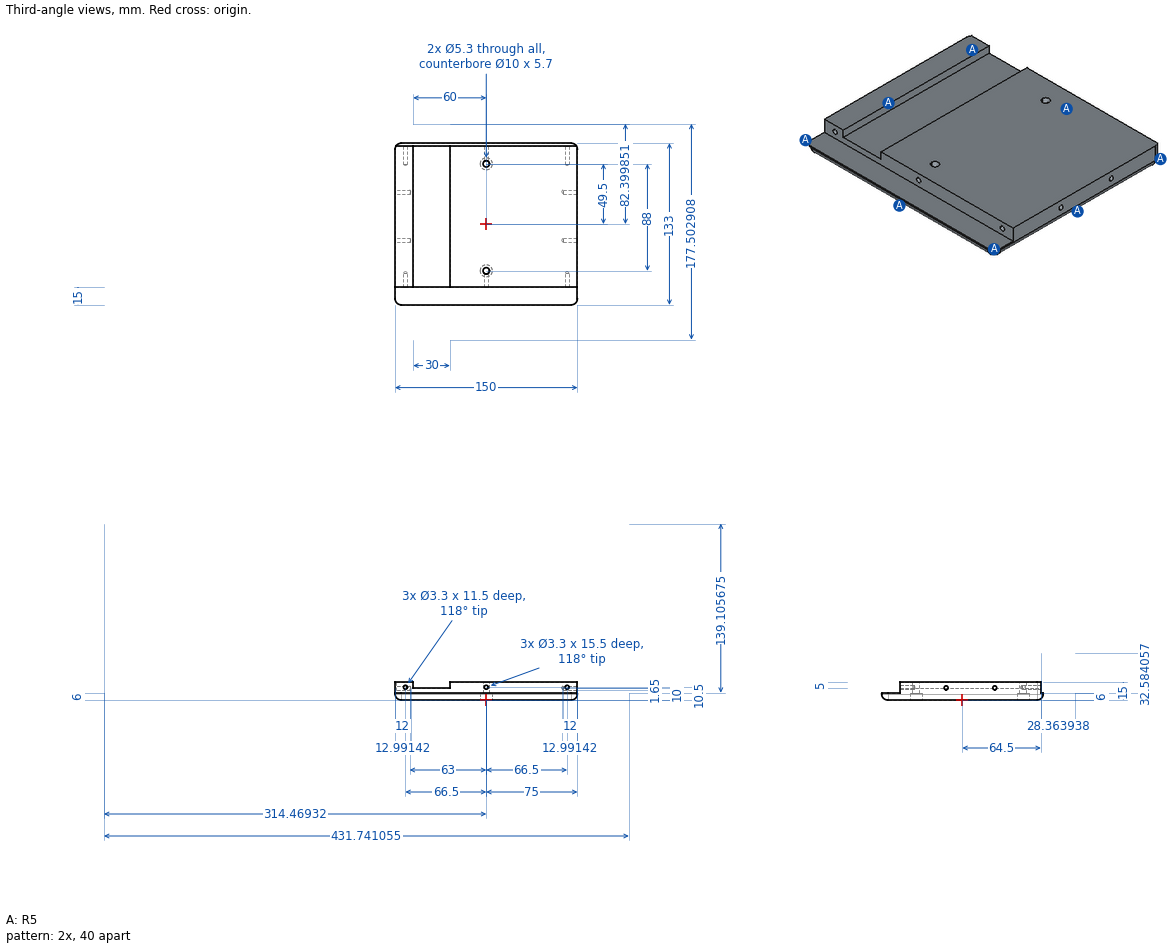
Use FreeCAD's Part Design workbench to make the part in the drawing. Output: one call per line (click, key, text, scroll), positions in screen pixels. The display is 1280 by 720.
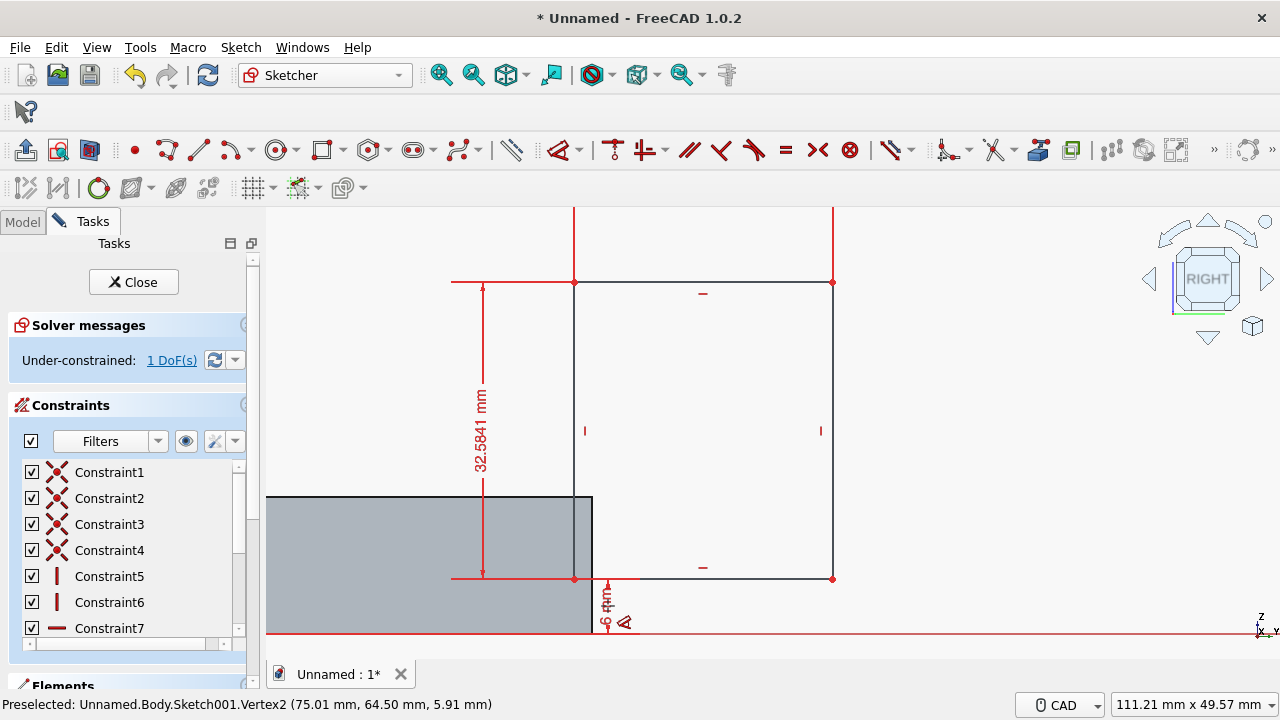
click(574, 282)
click(434, 248)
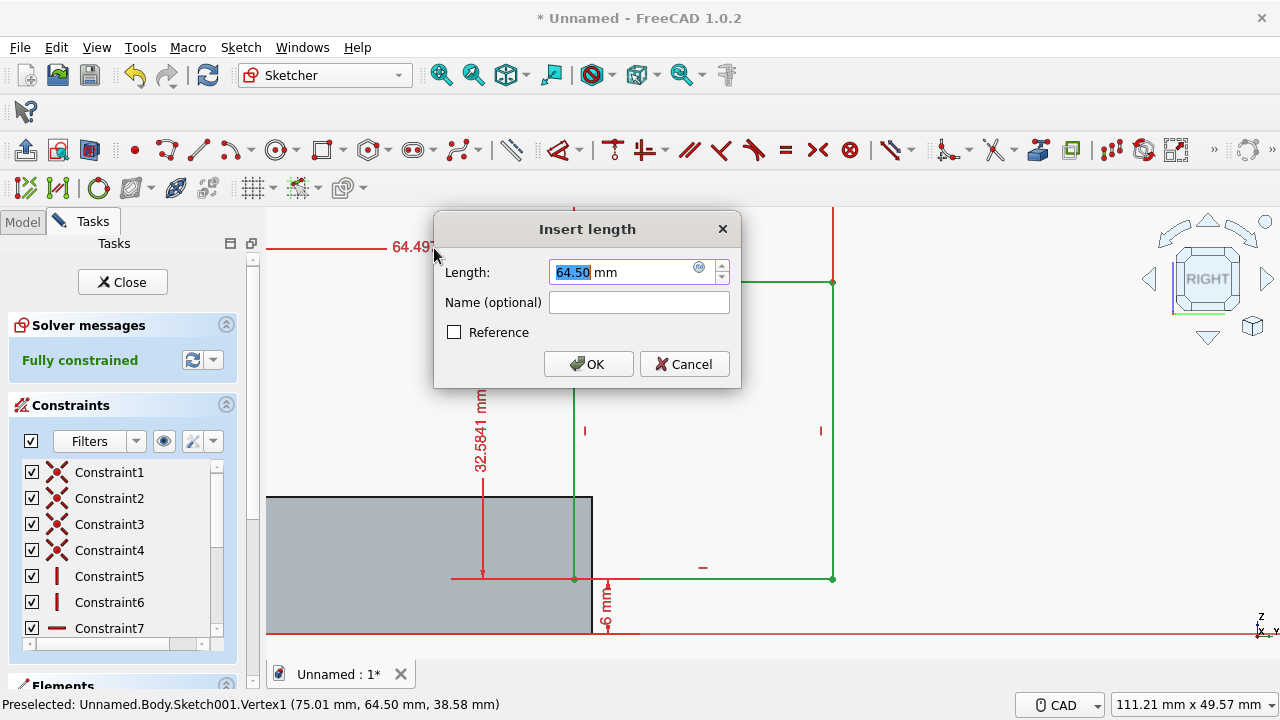
text(64.5)
key(Return)
key(Escape)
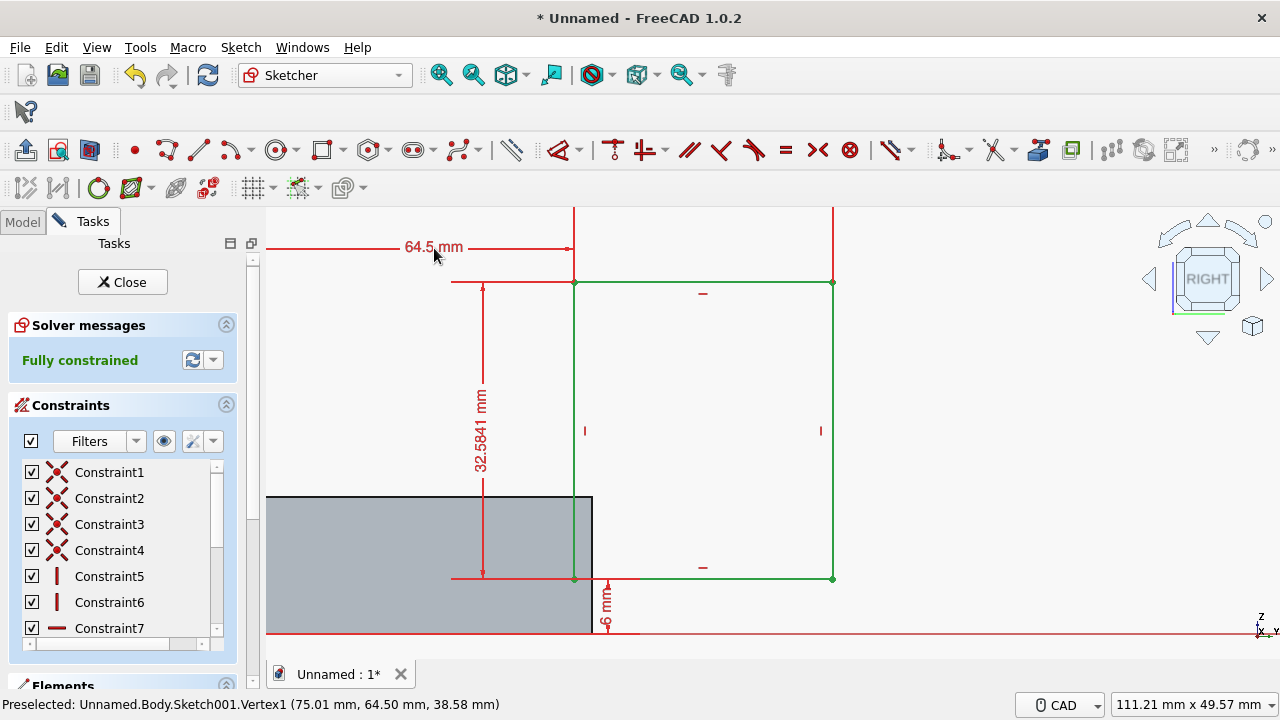
click(123, 282)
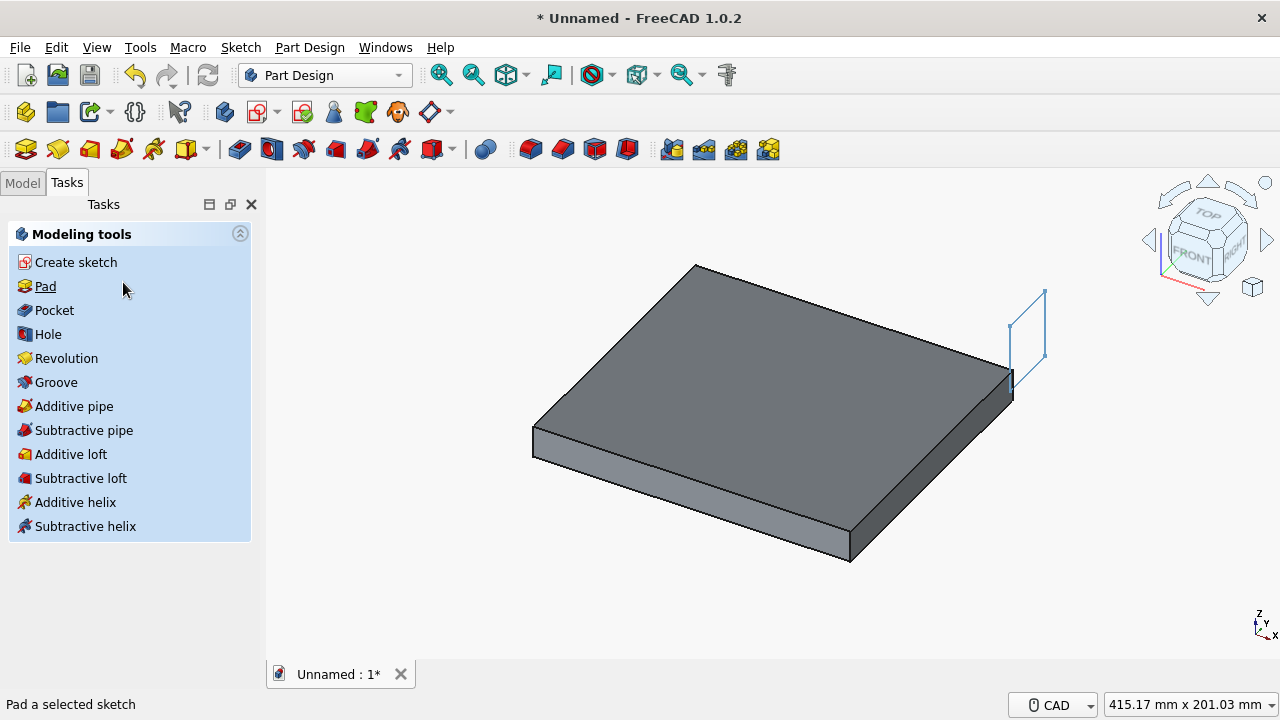
click(240, 150)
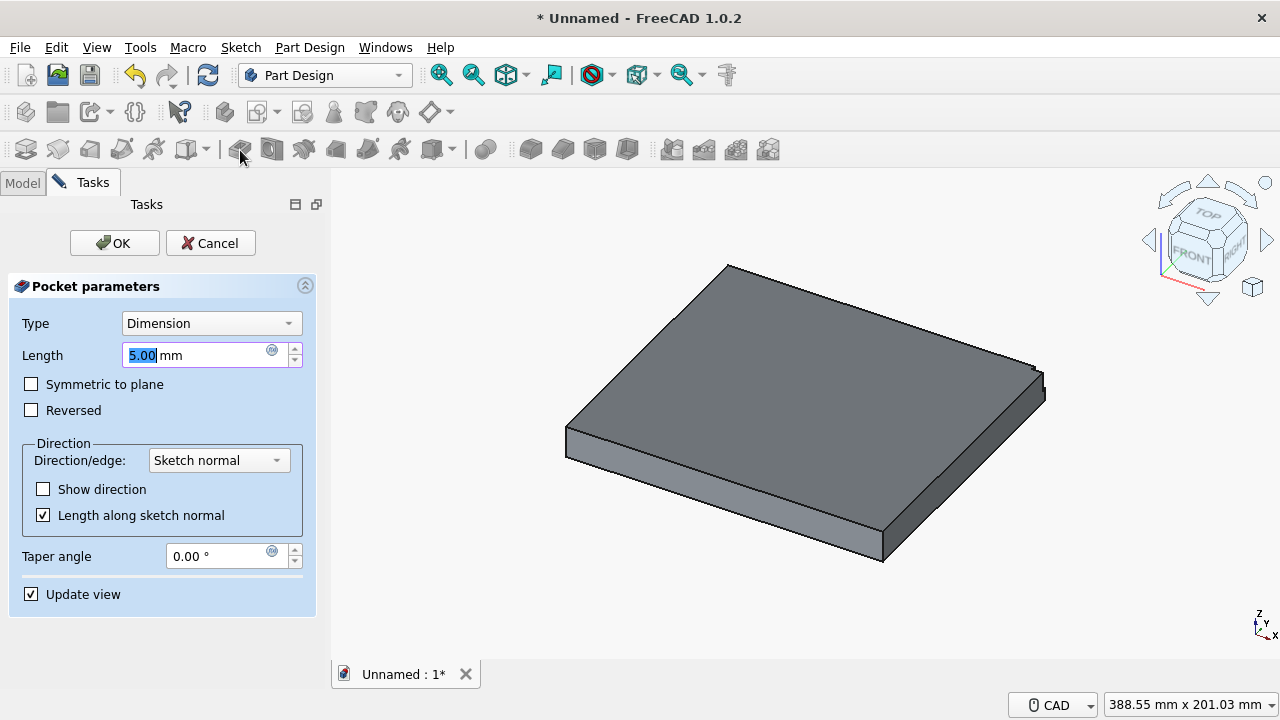
click(212, 324)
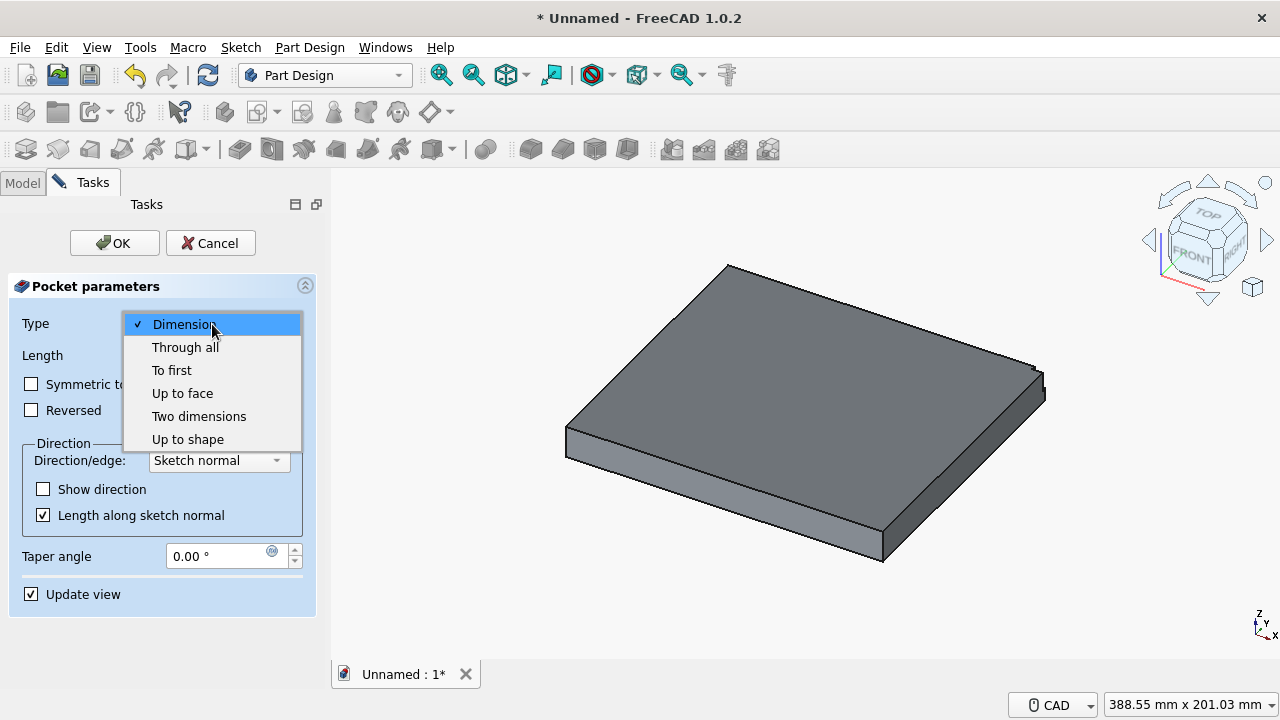
click(212, 348)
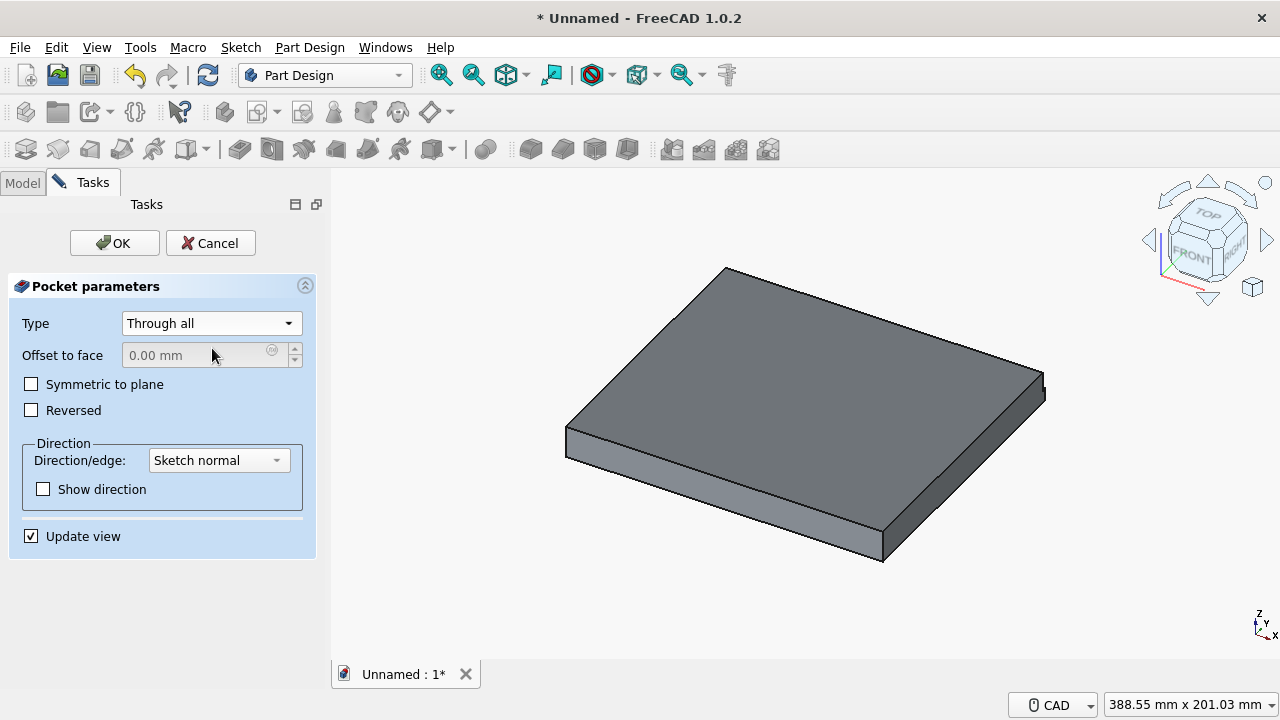
click(115, 243)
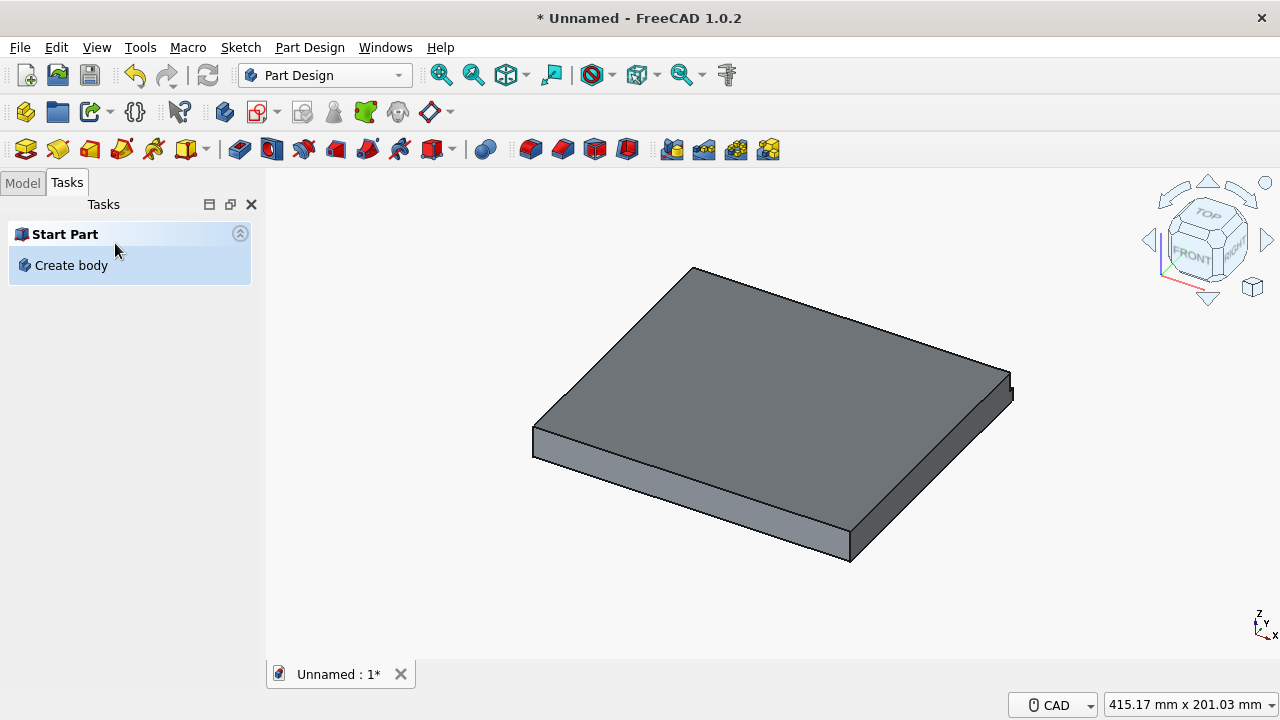
click(850, 546)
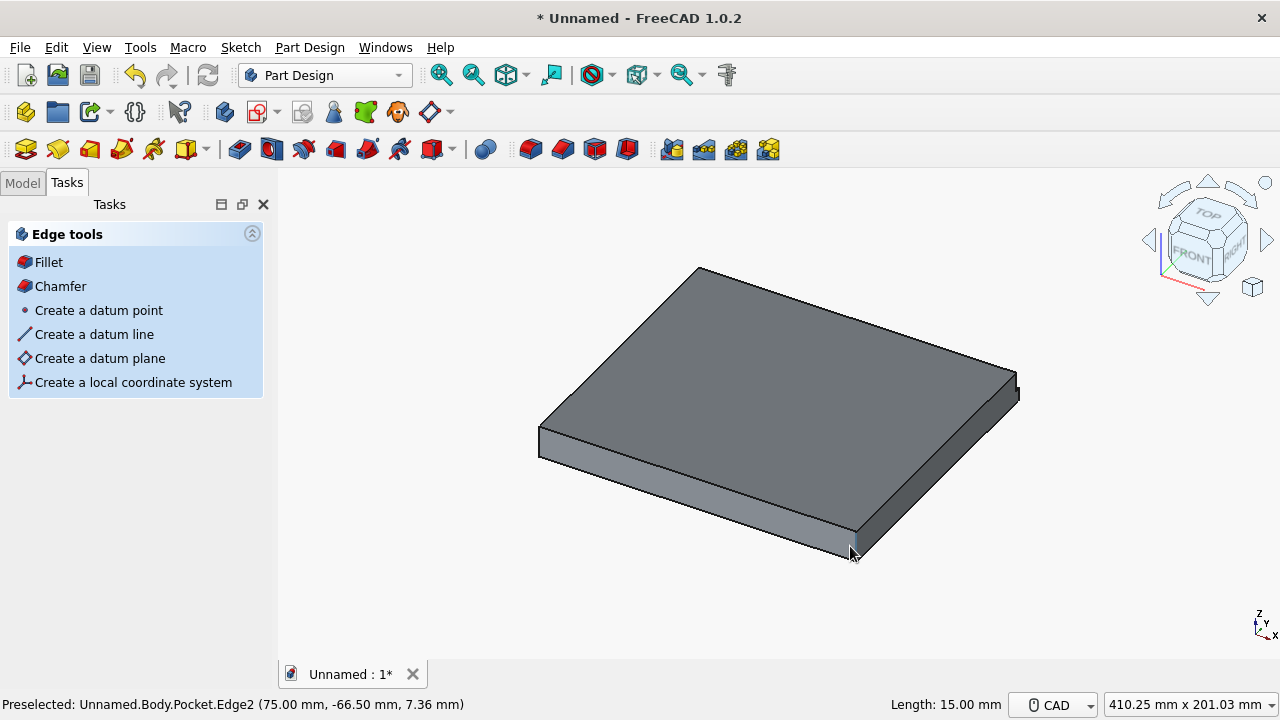
key(0)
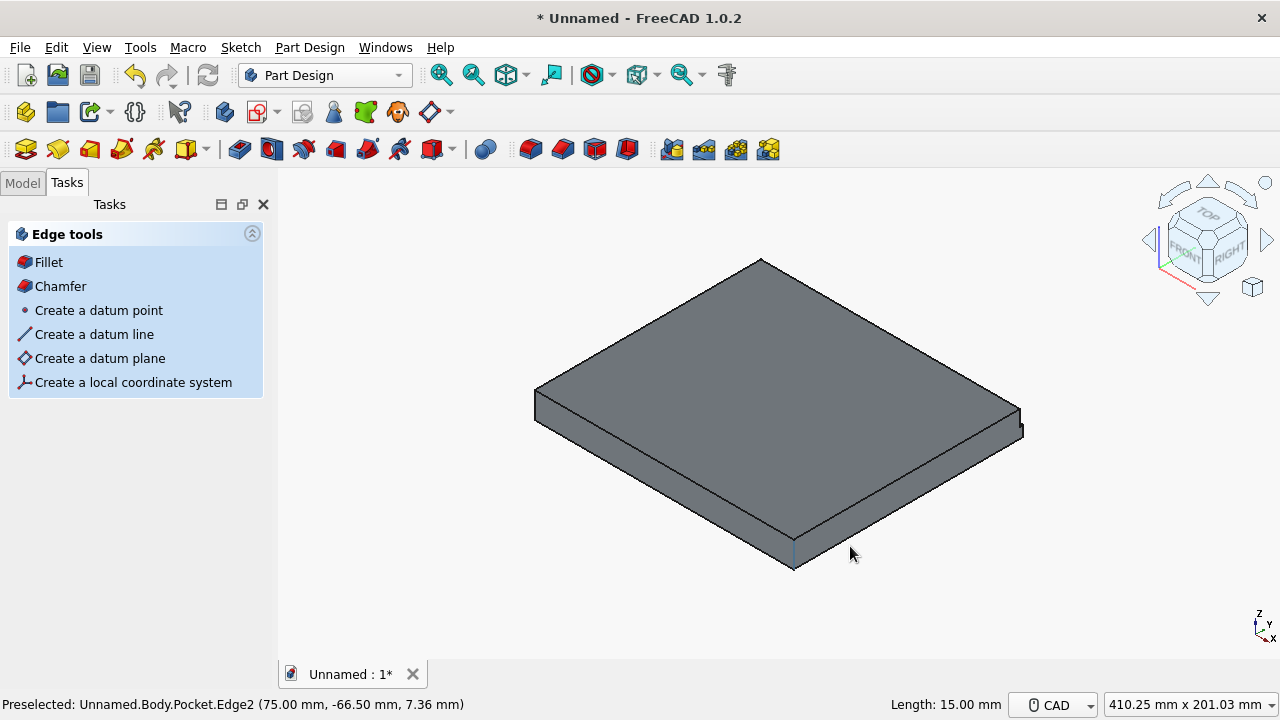
key(2)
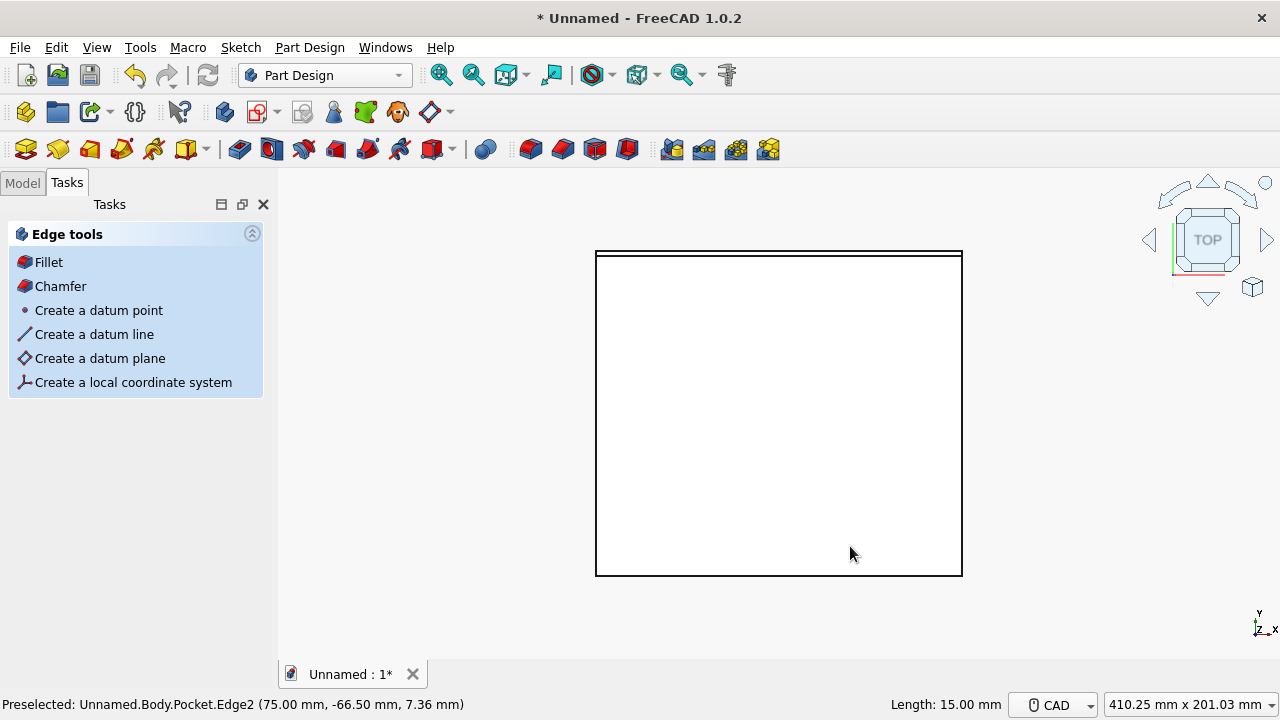
key(1)